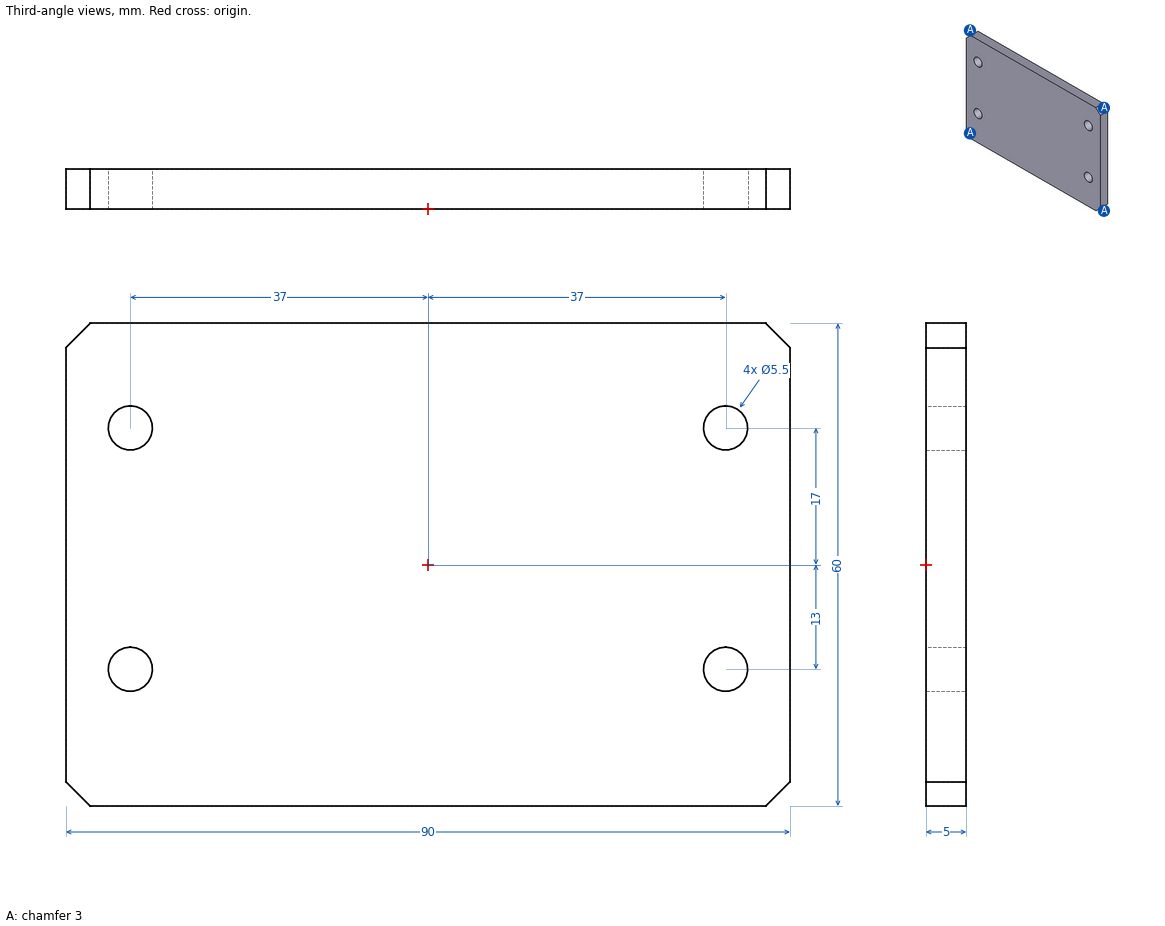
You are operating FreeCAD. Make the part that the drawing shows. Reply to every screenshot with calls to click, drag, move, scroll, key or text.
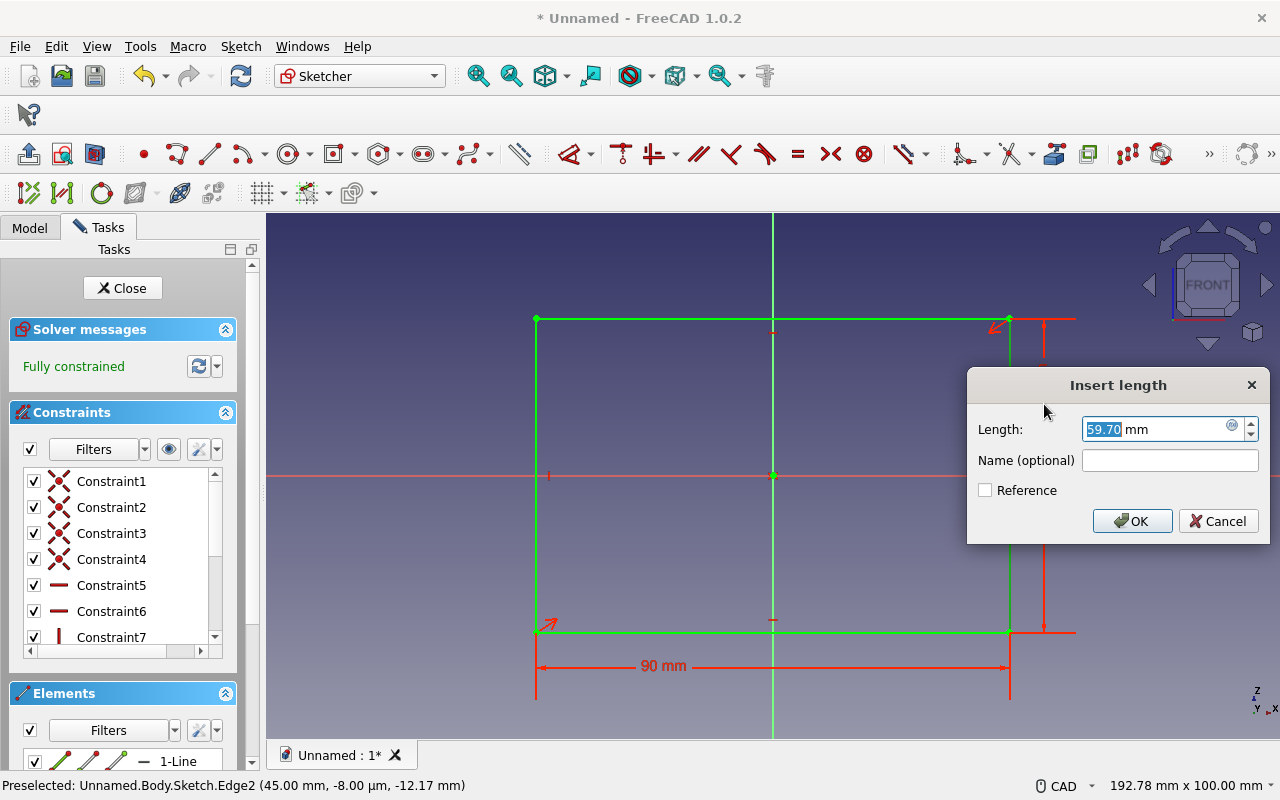
text(60)
key(Return)
key(Escape)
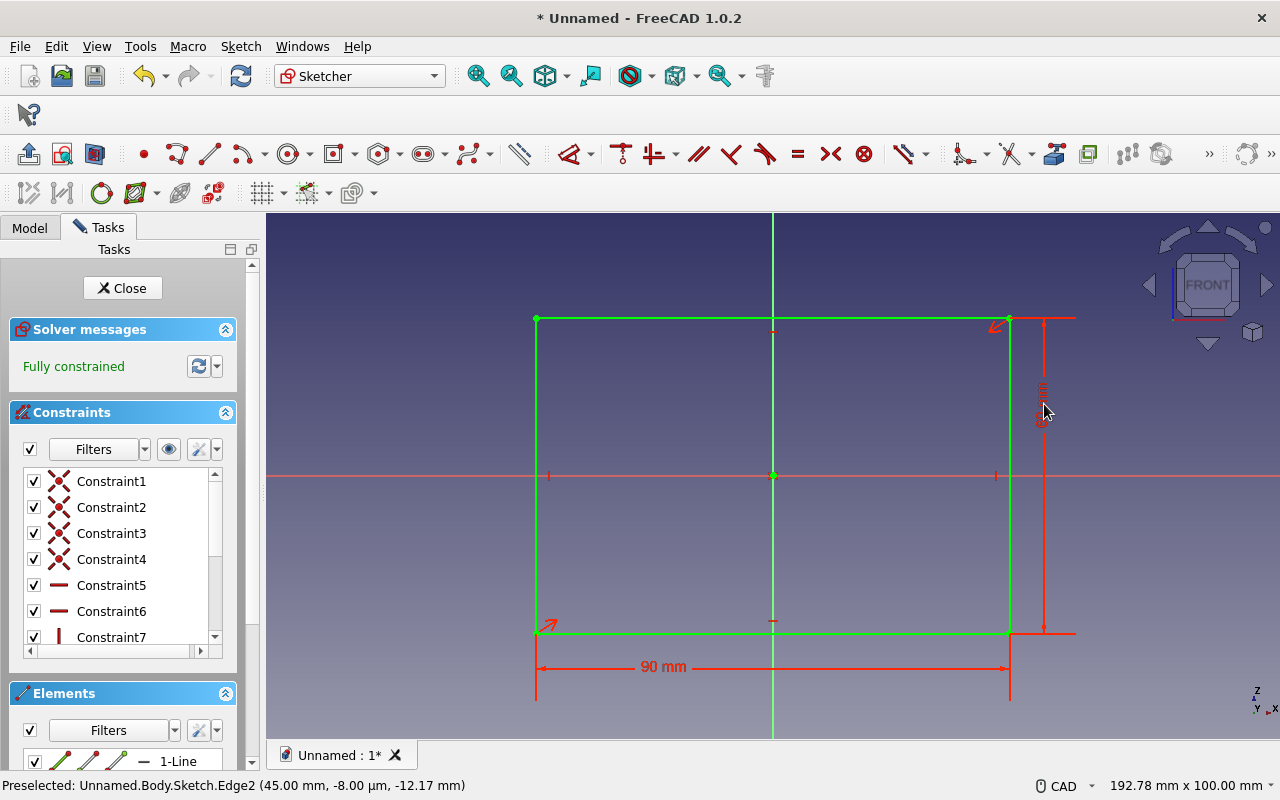
click(123, 288)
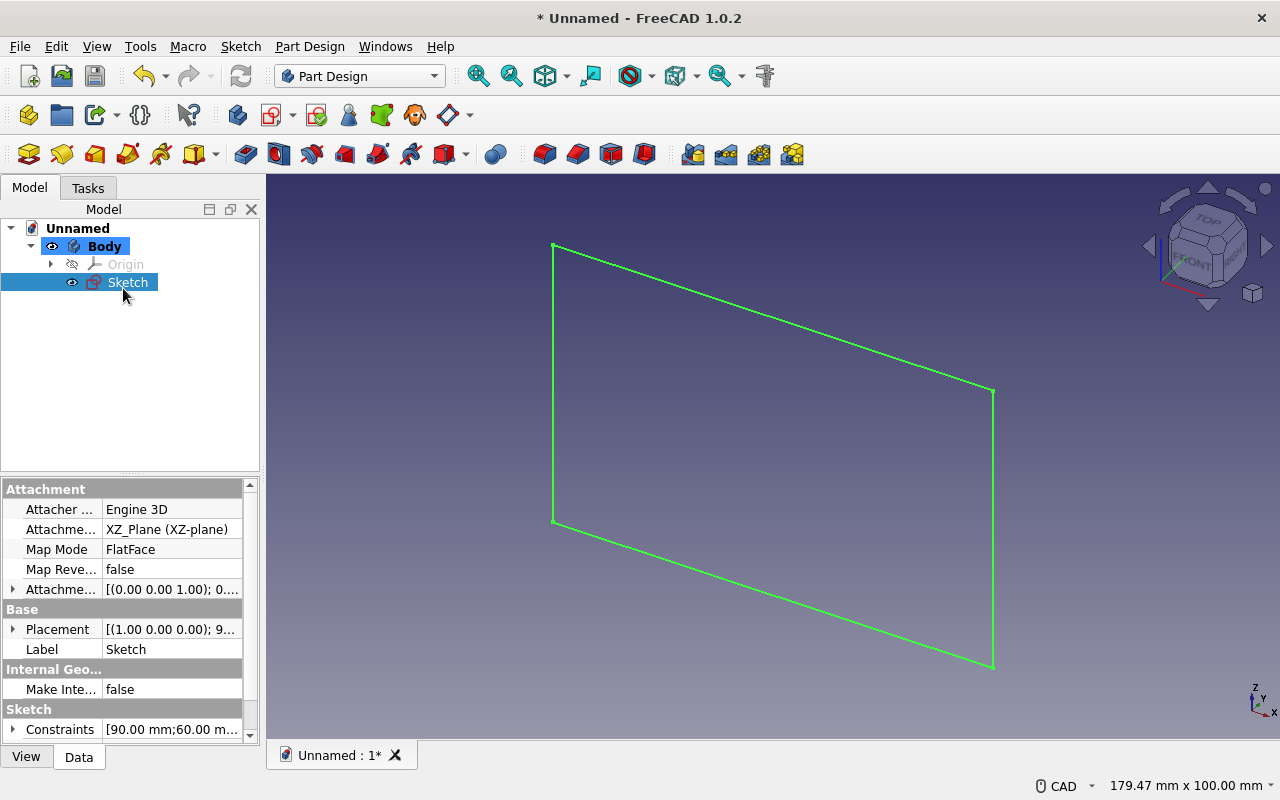
click(29, 154)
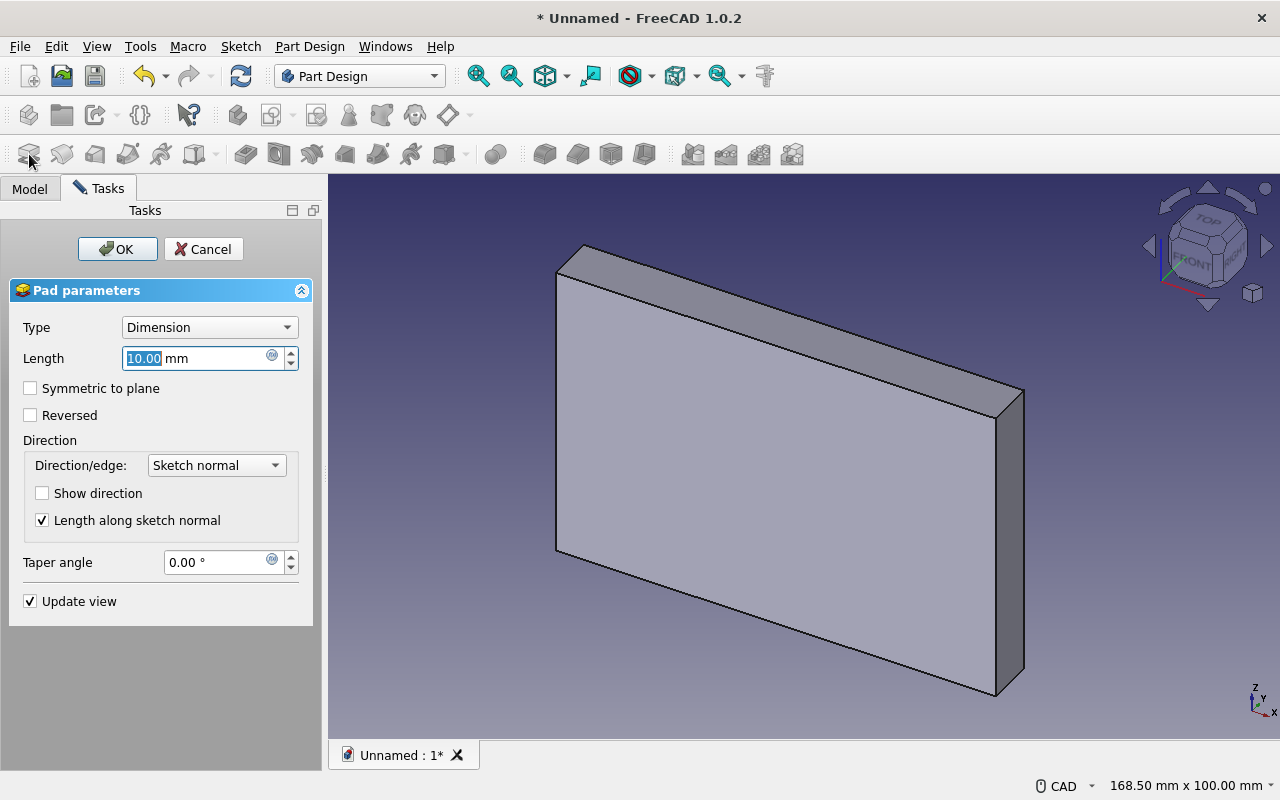
text(5)
key(Tab)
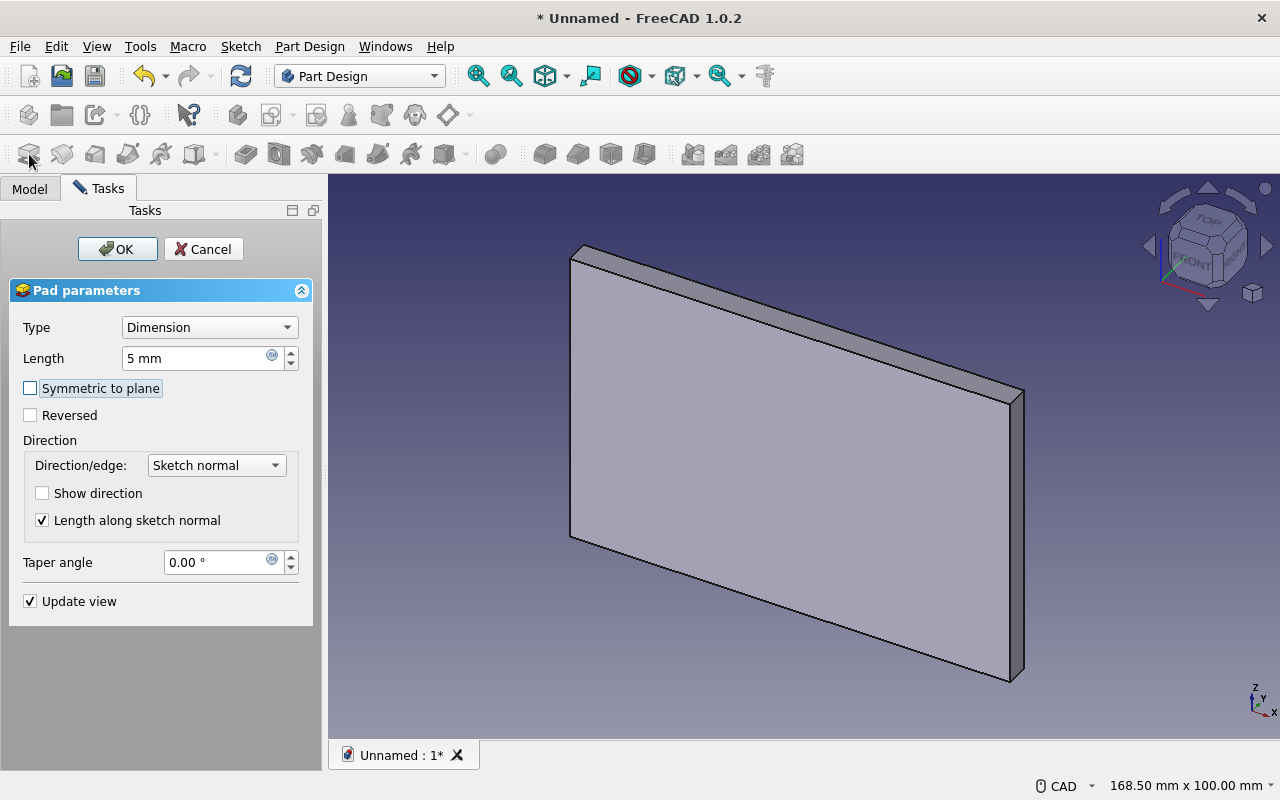
click(31, 415)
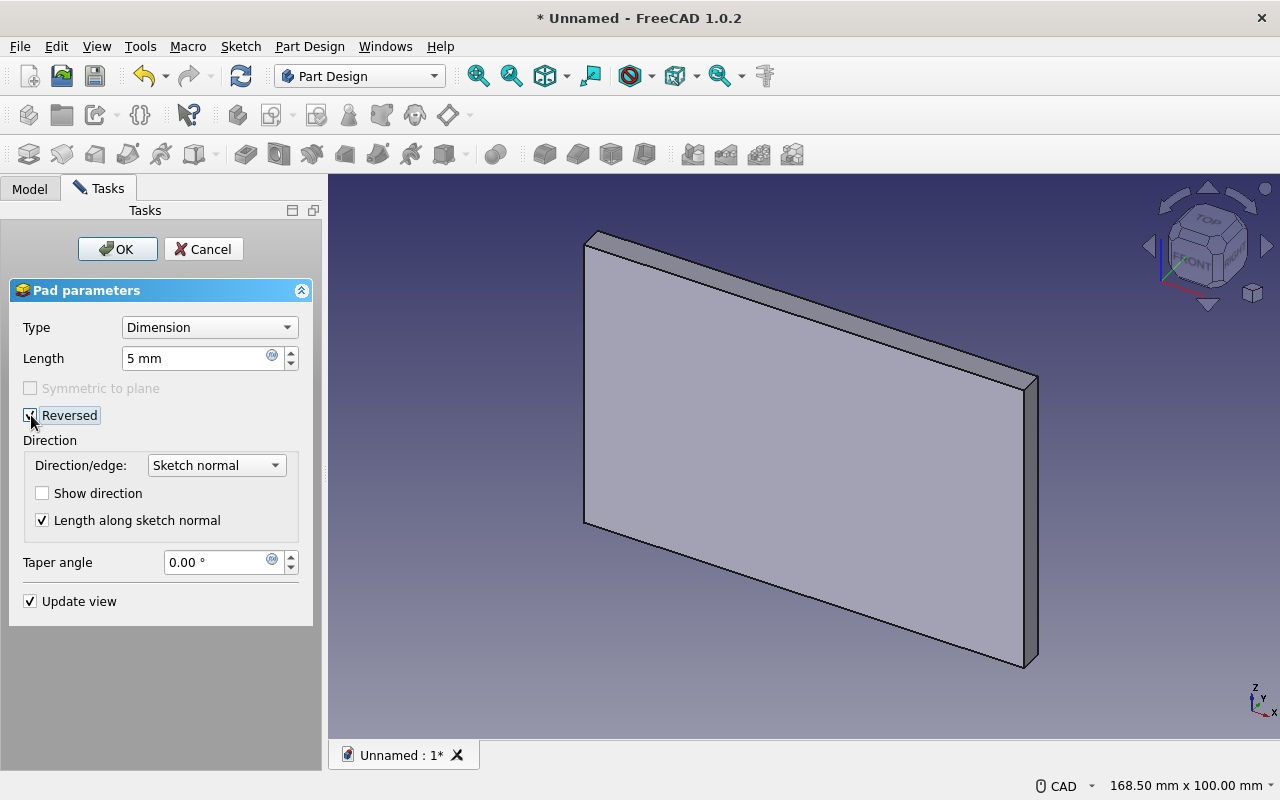
click(118, 249)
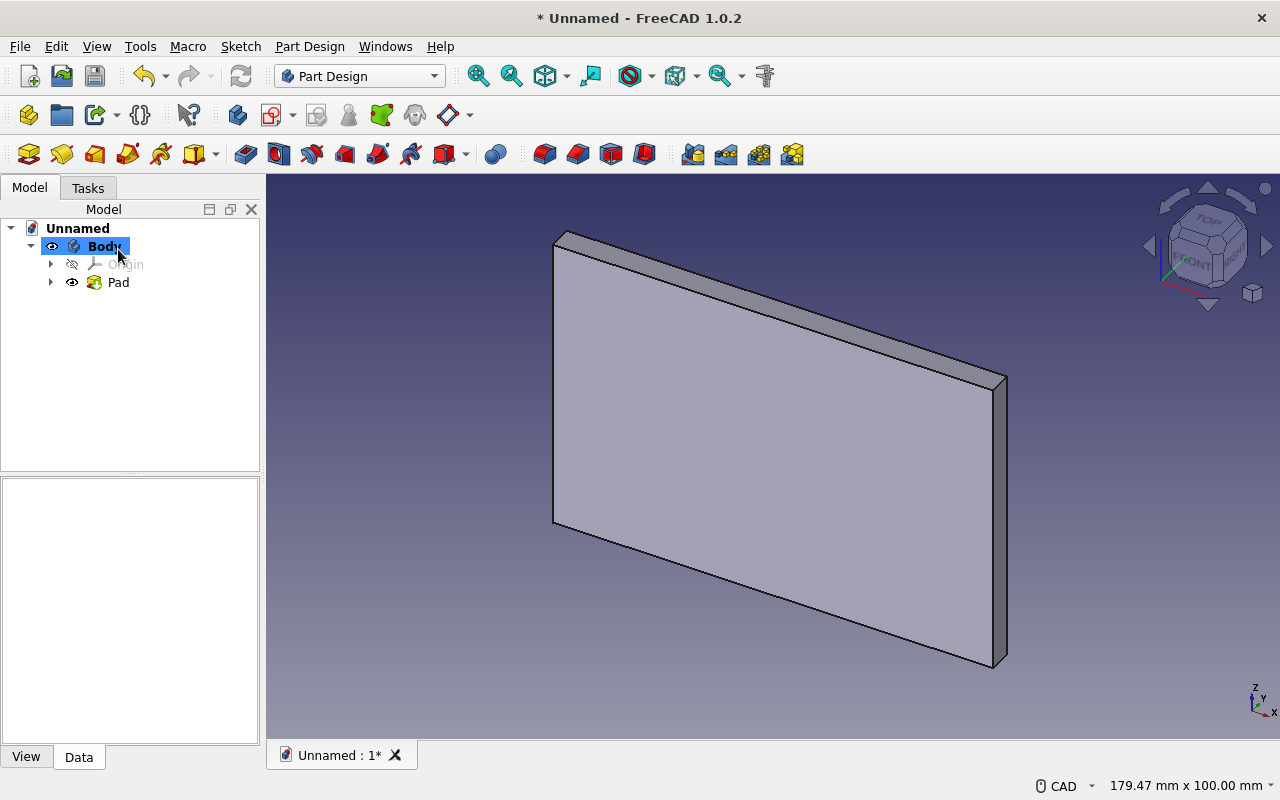
click(1000, 383)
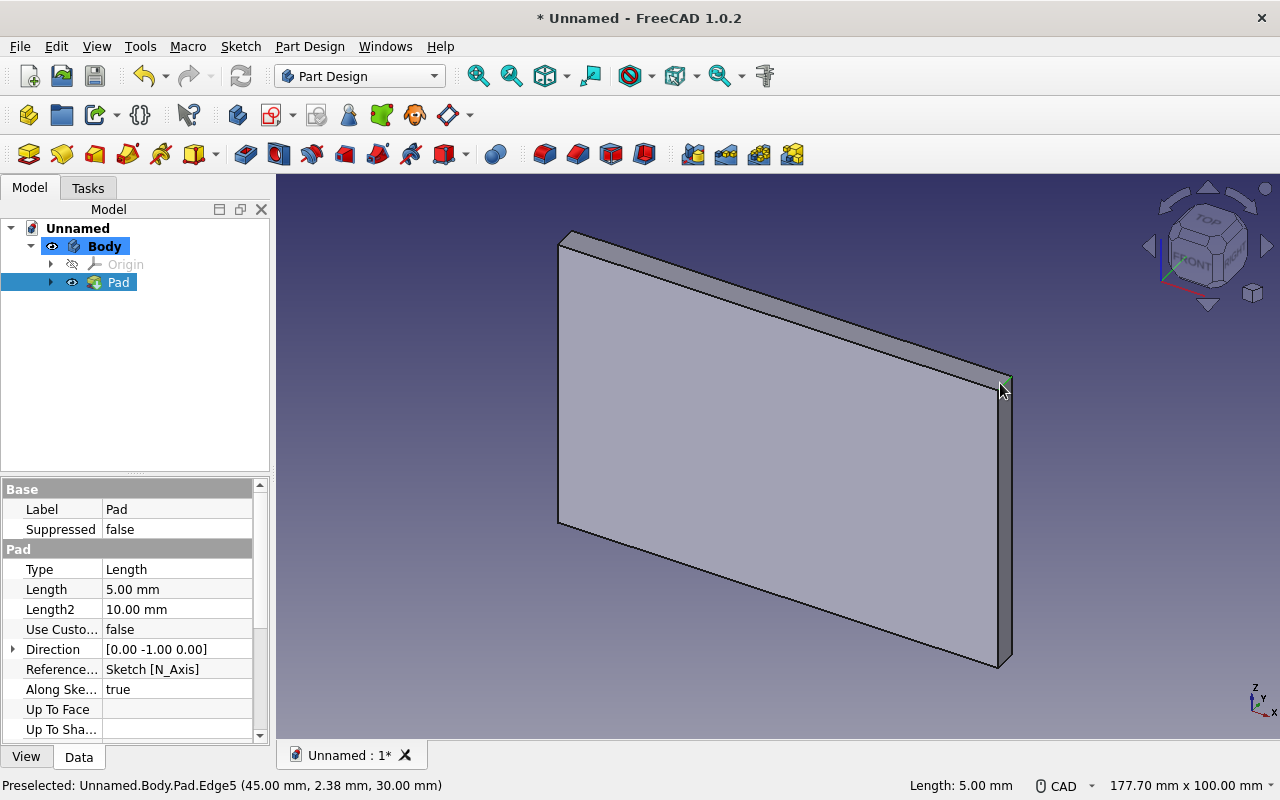
key(0)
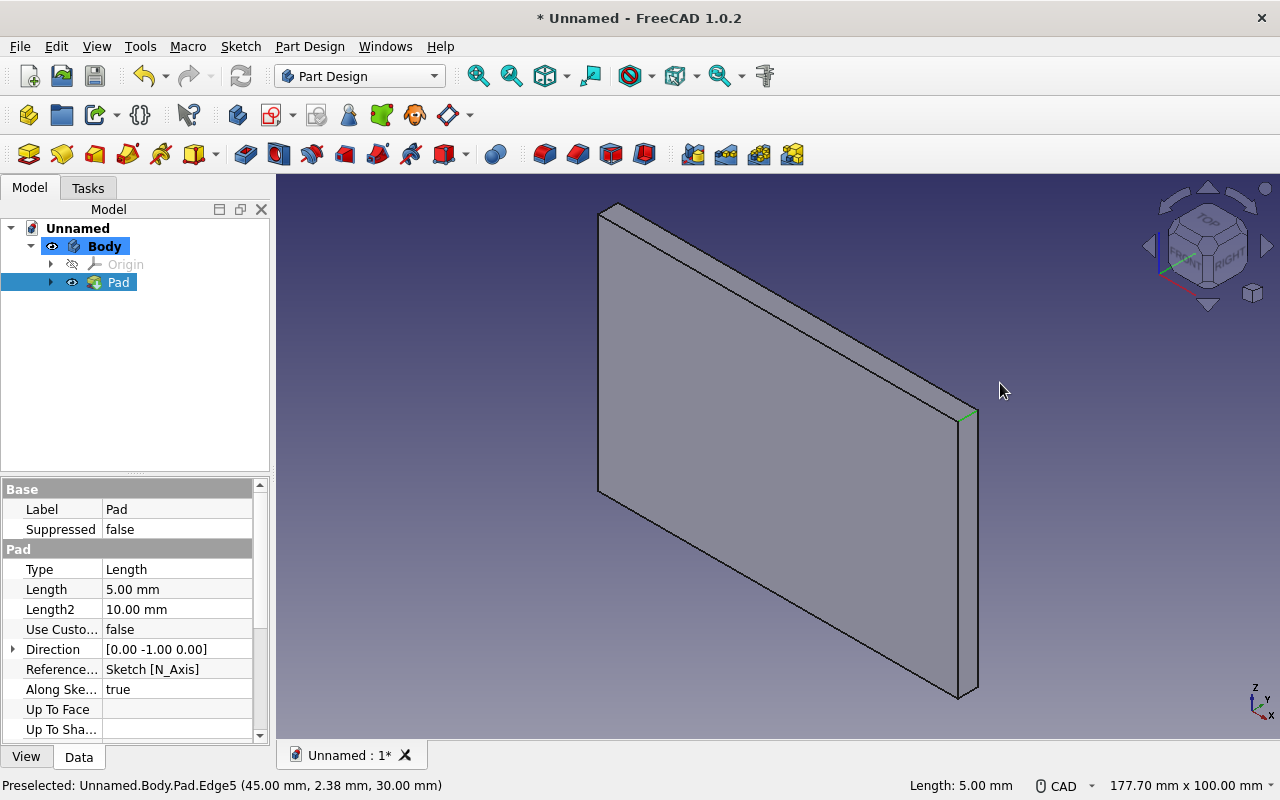
key(2)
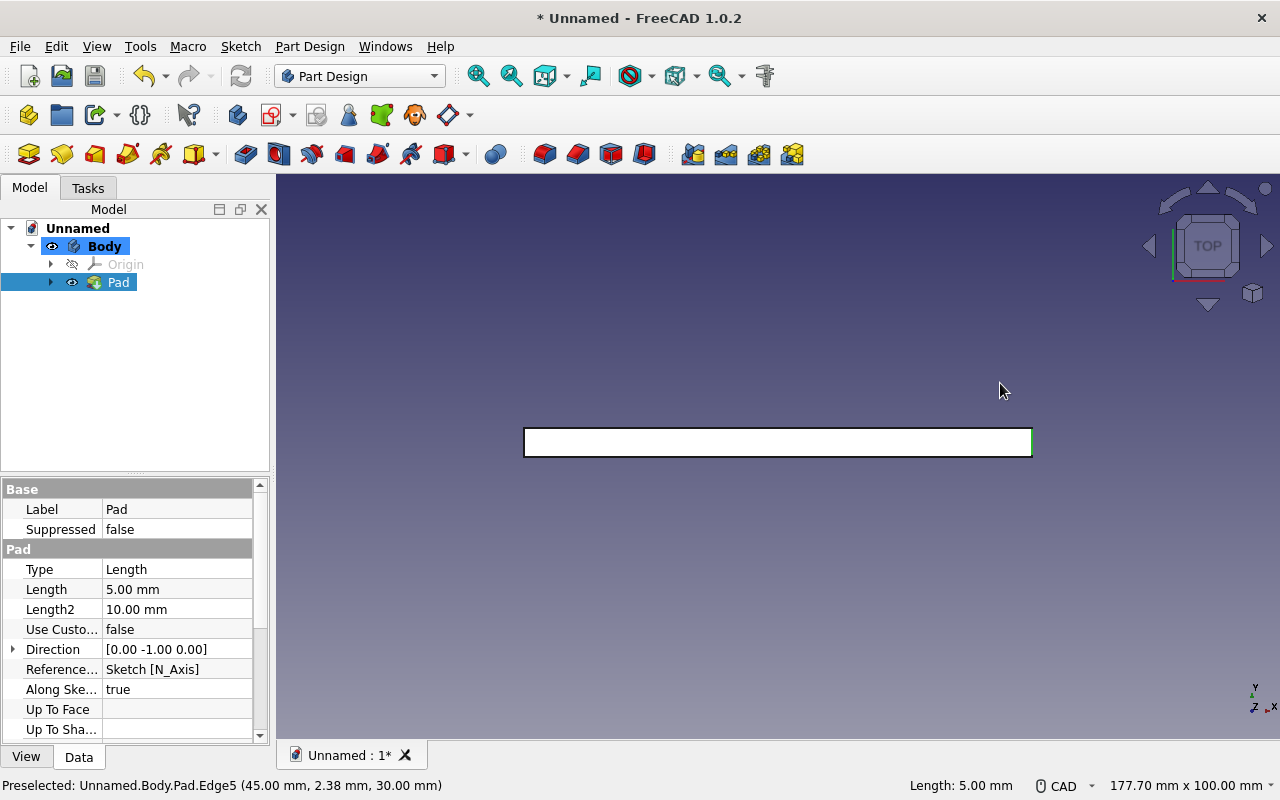
click(524, 441, ctrl)